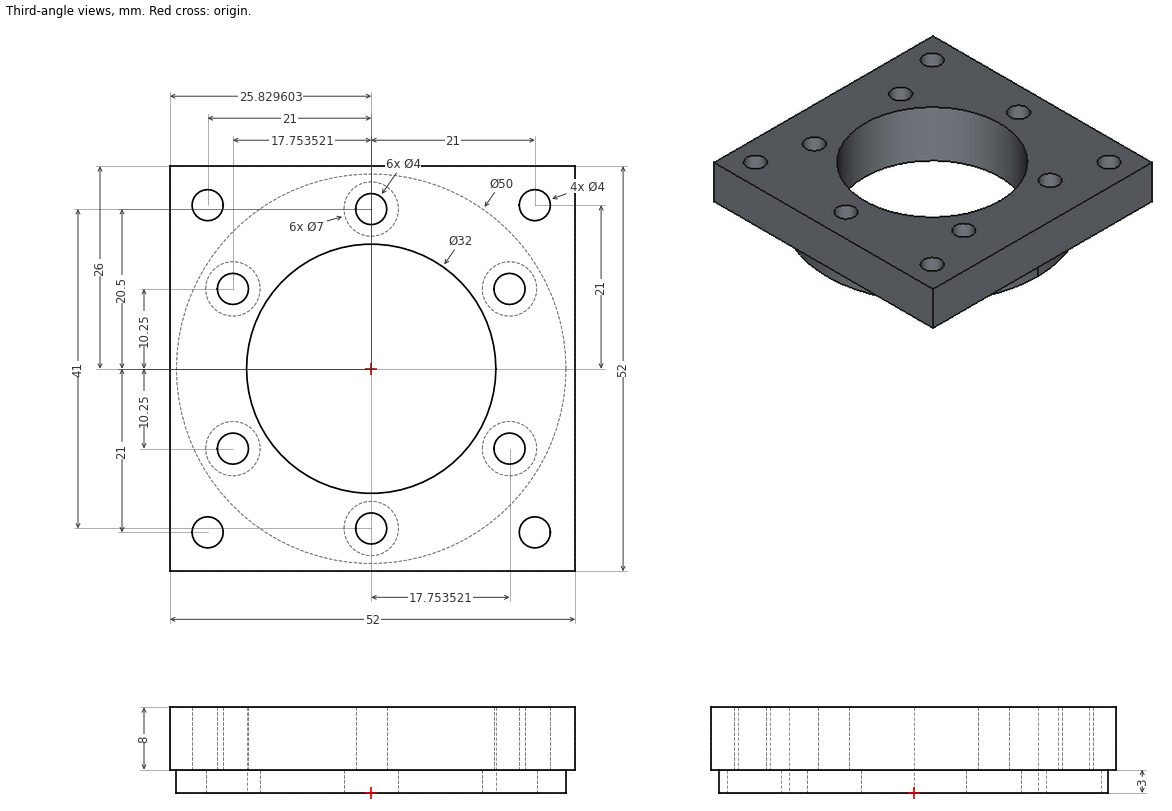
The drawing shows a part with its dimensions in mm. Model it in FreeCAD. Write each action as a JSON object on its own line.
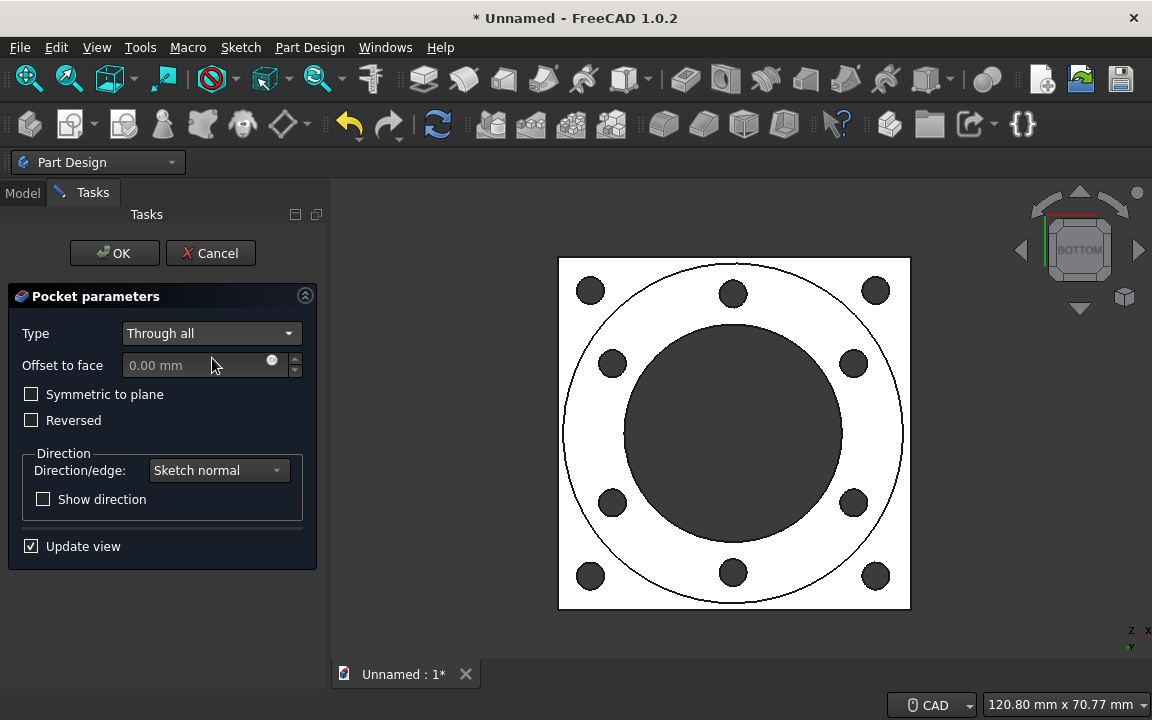
{"action": "left_click", "coordinate": [115, 253]}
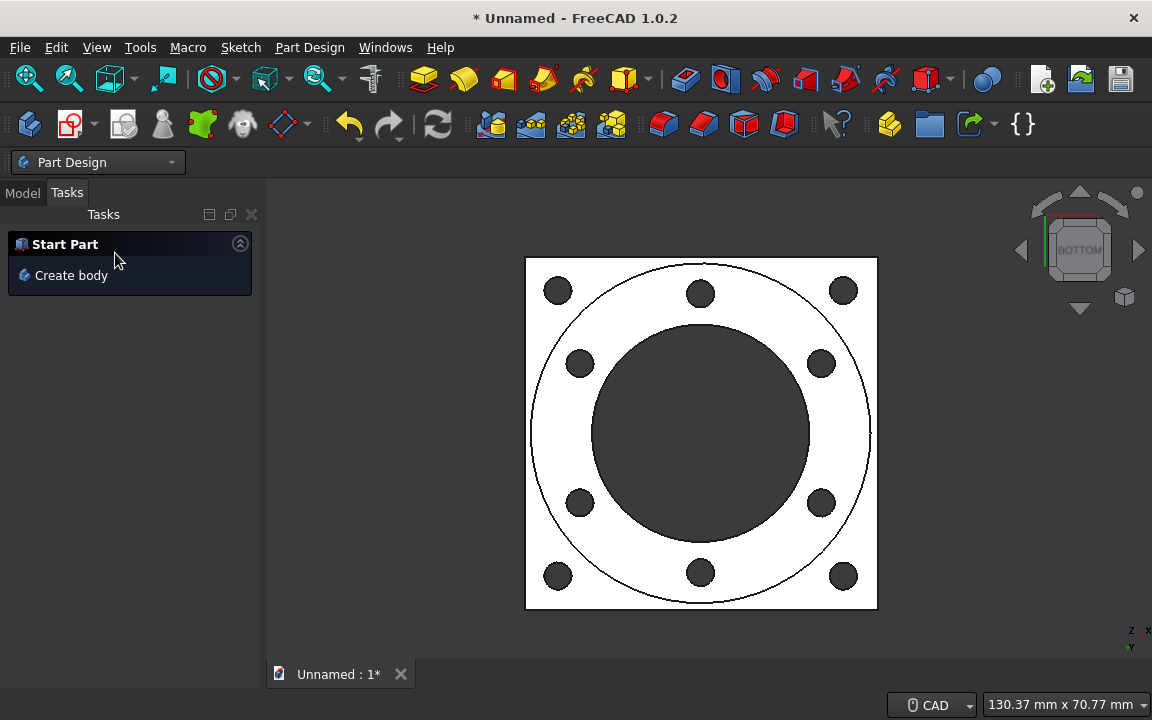
{"action": "left_click", "coordinate": [70, 124]}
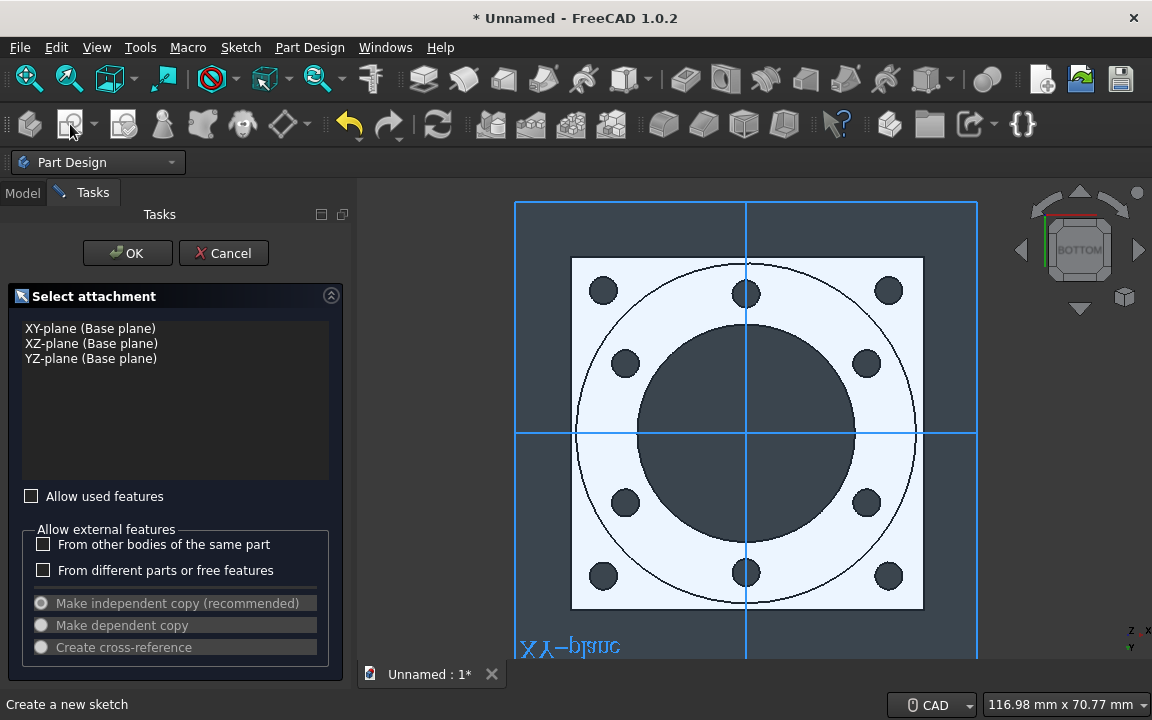
{"action": "left_click", "coordinate": [82, 328]}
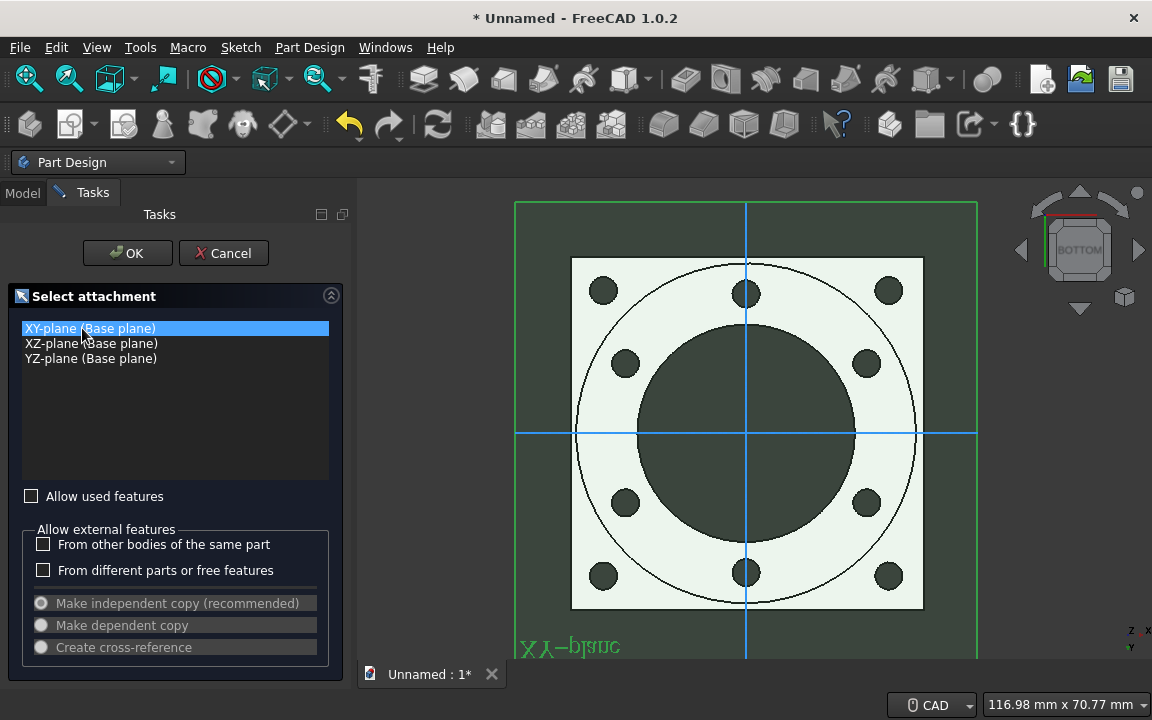
{"action": "left_click", "coordinate": [128, 253]}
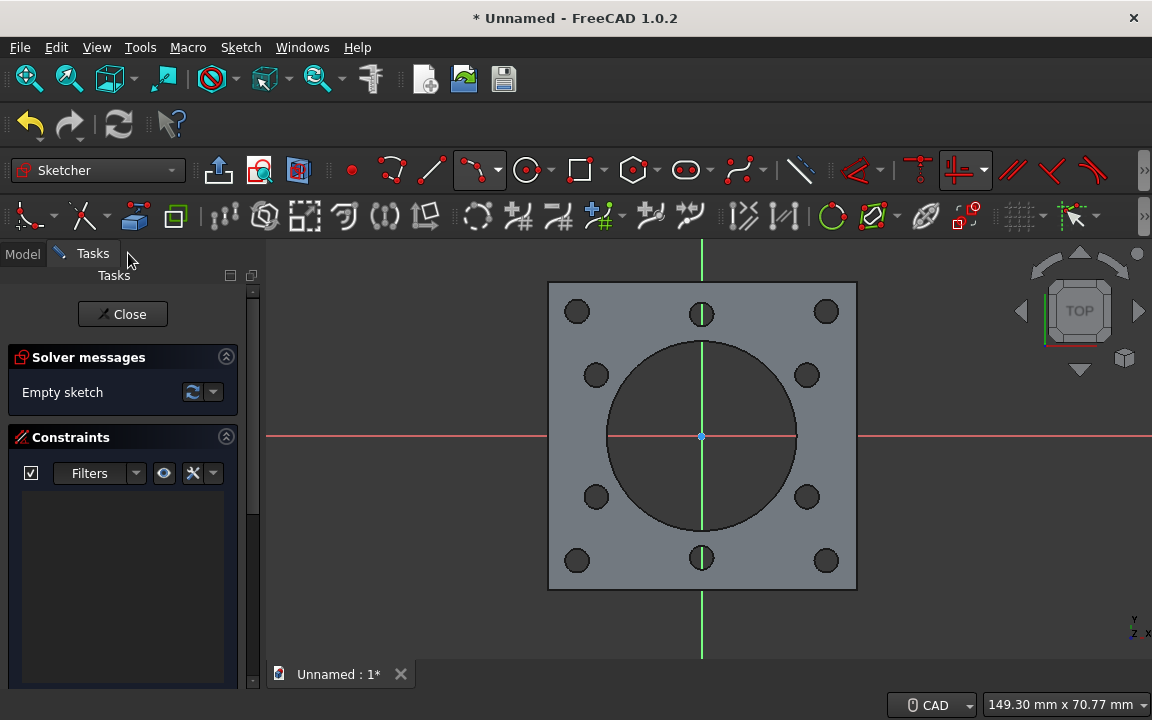
{"action": "key", "text": "q s"}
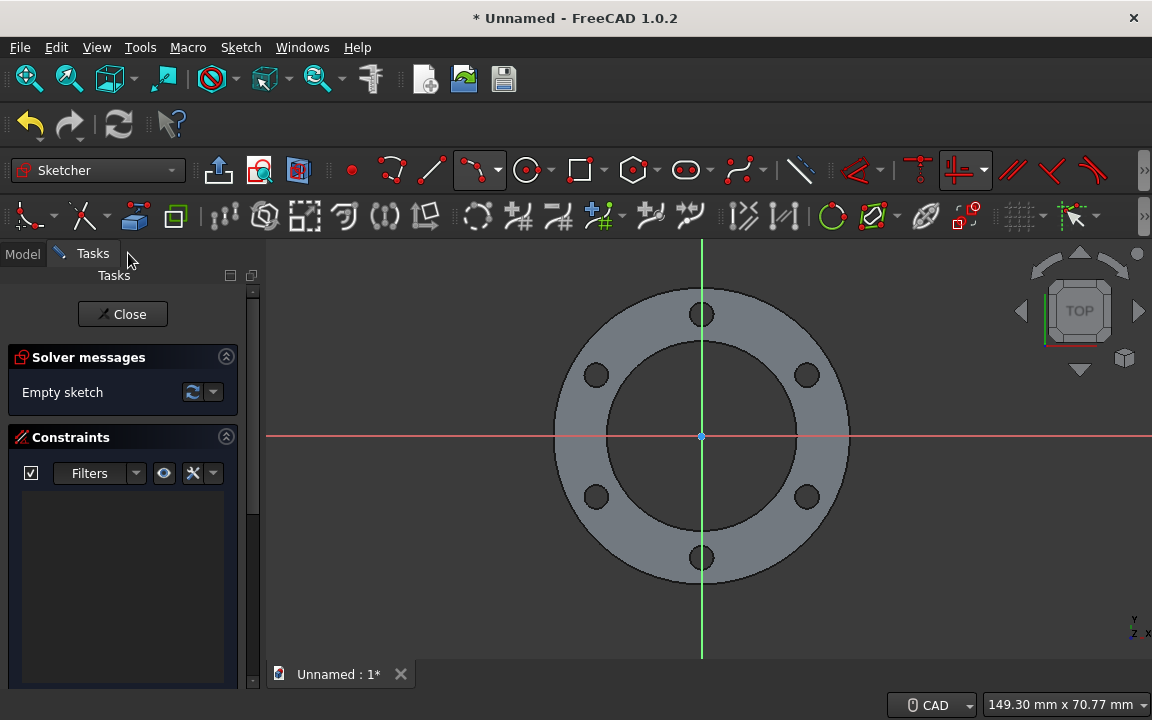
{"action": "key", "text": "g c"}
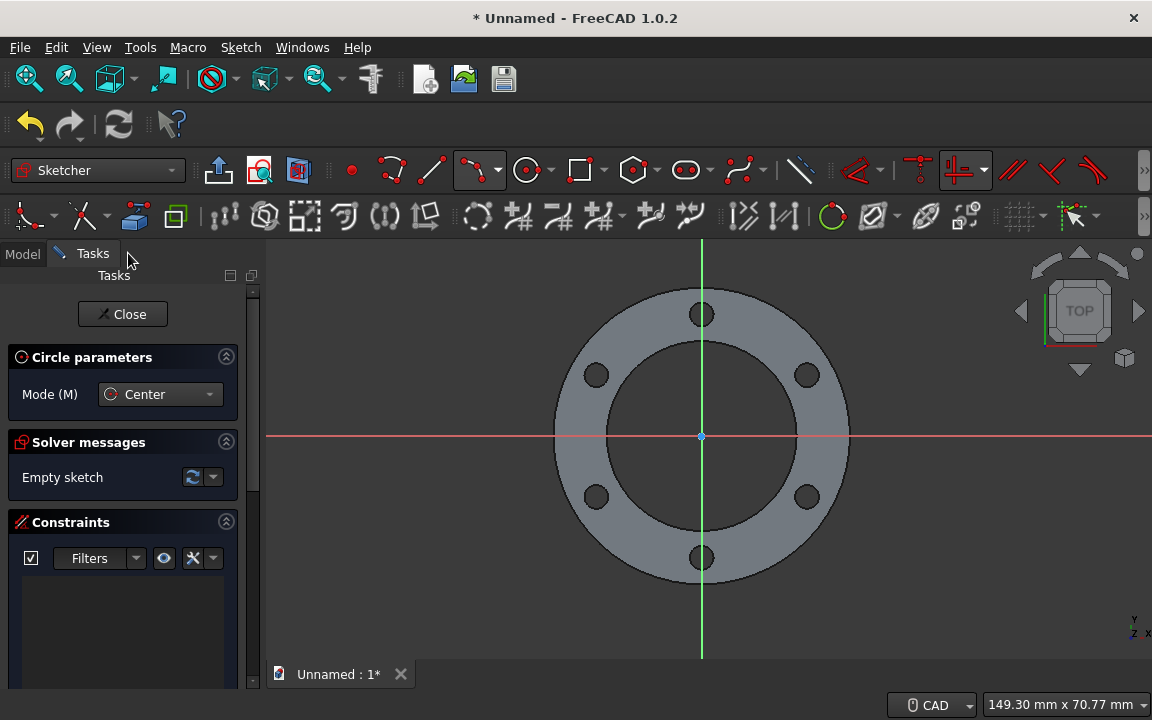
{"action": "left_click", "coordinate": [702, 314]}
{"action": "mouse_move", "coordinate": [716, 300]}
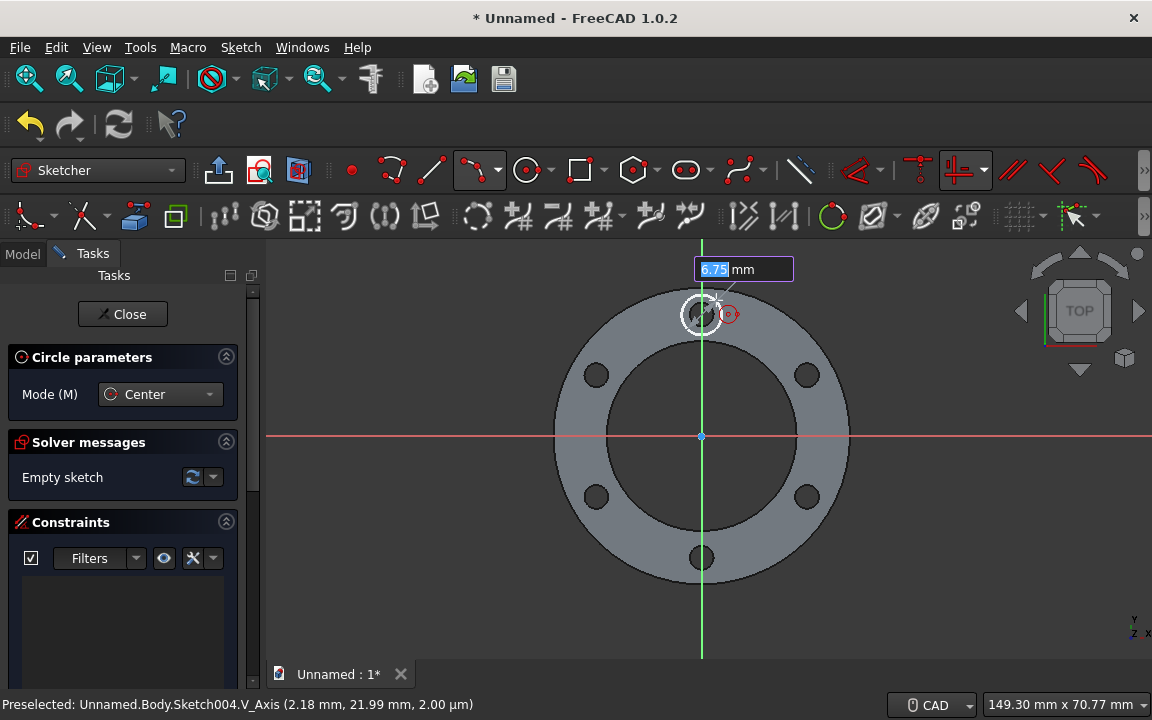
{"action": "type", "text": "7"}
{"action": "key", "text": "Return"}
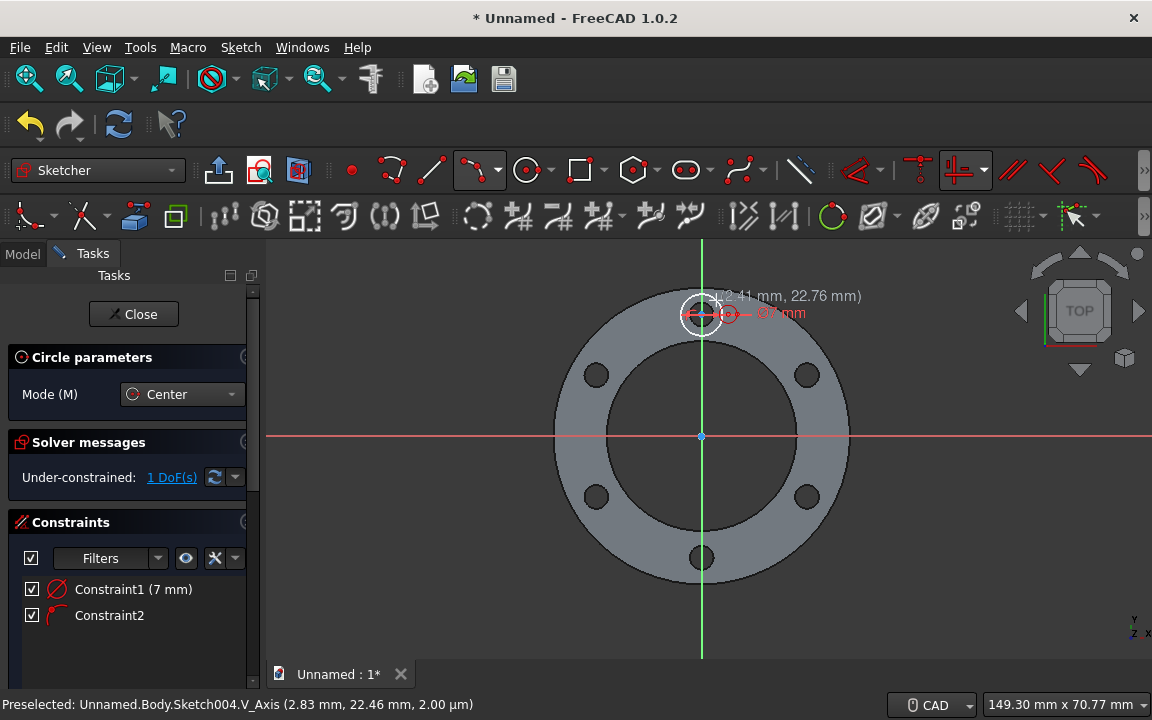
{"action": "left_click", "coordinate": [596, 375]}
{"action": "mouse_move", "coordinate": [611, 361]}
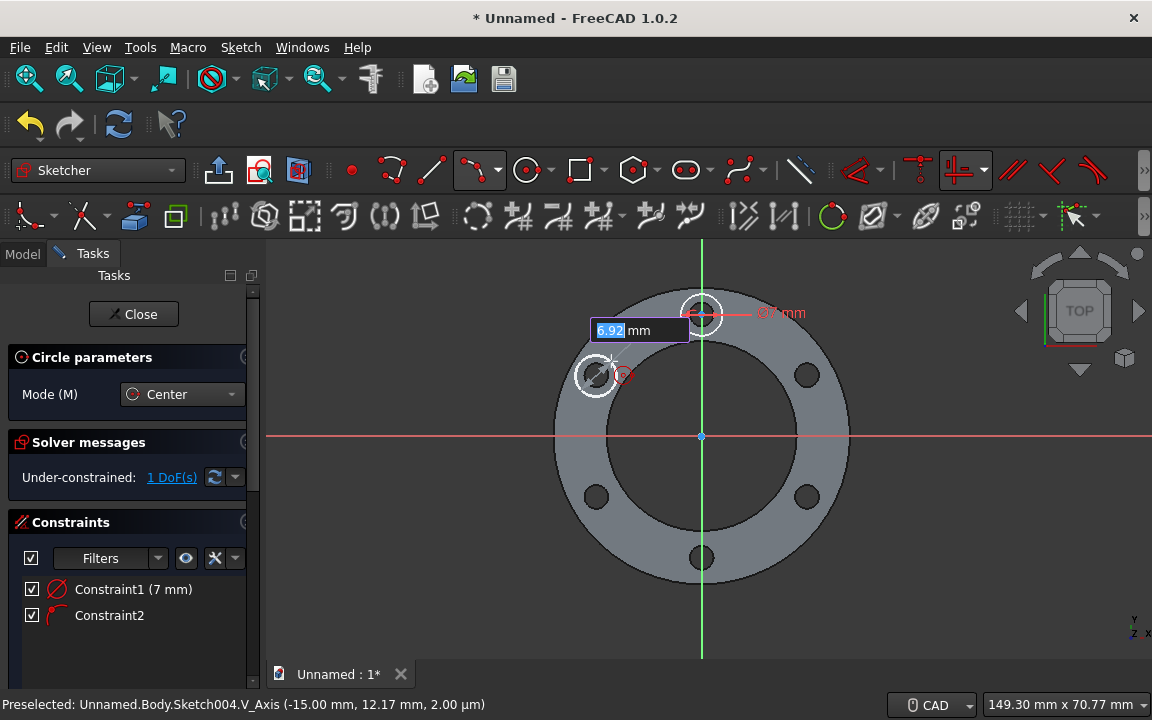
{"action": "type", "text": "7"}
{"action": "key", "text": "Return"}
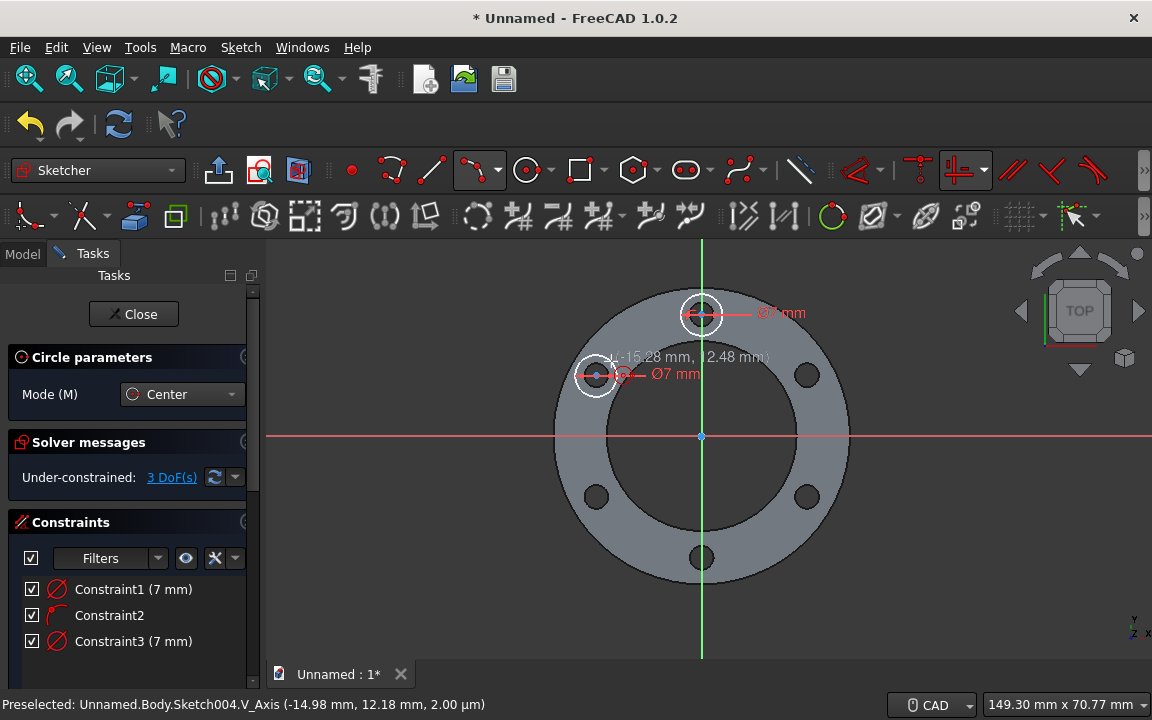
{"action": "left_click", "coordinate": [596, 497]}
{"action": "mouse_move", "coordinate": [611, 482]}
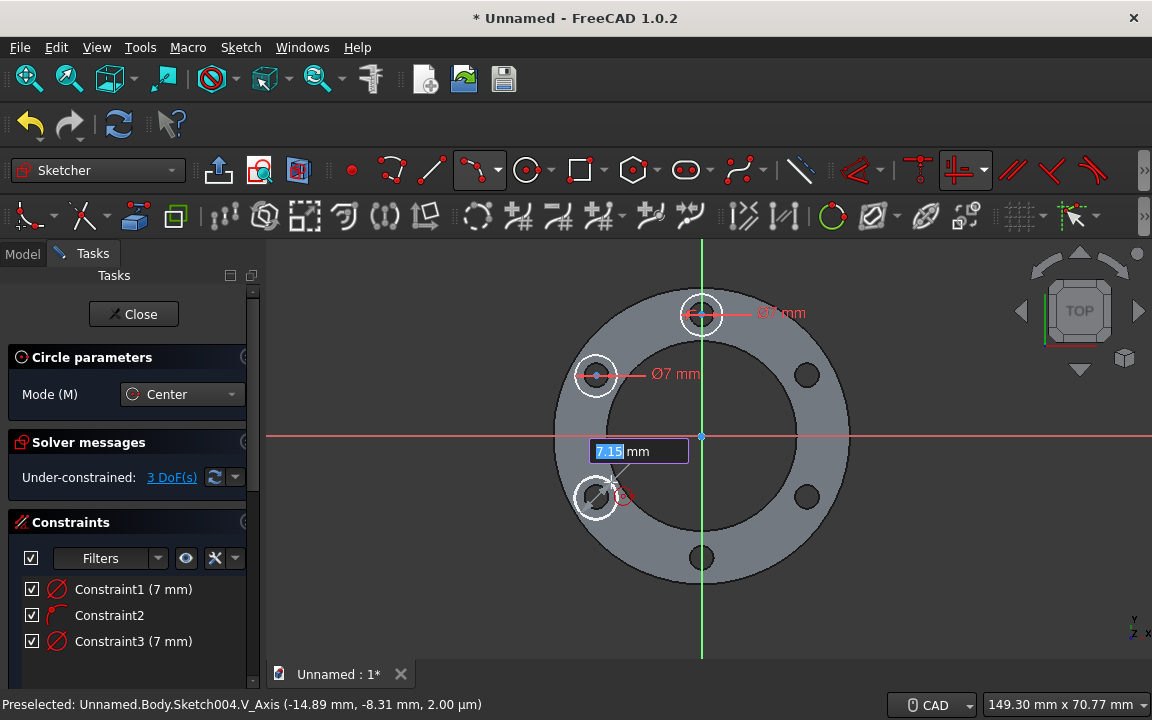
{"action": "type", "text": "7"}
{"action": "key", "text": "Return"}